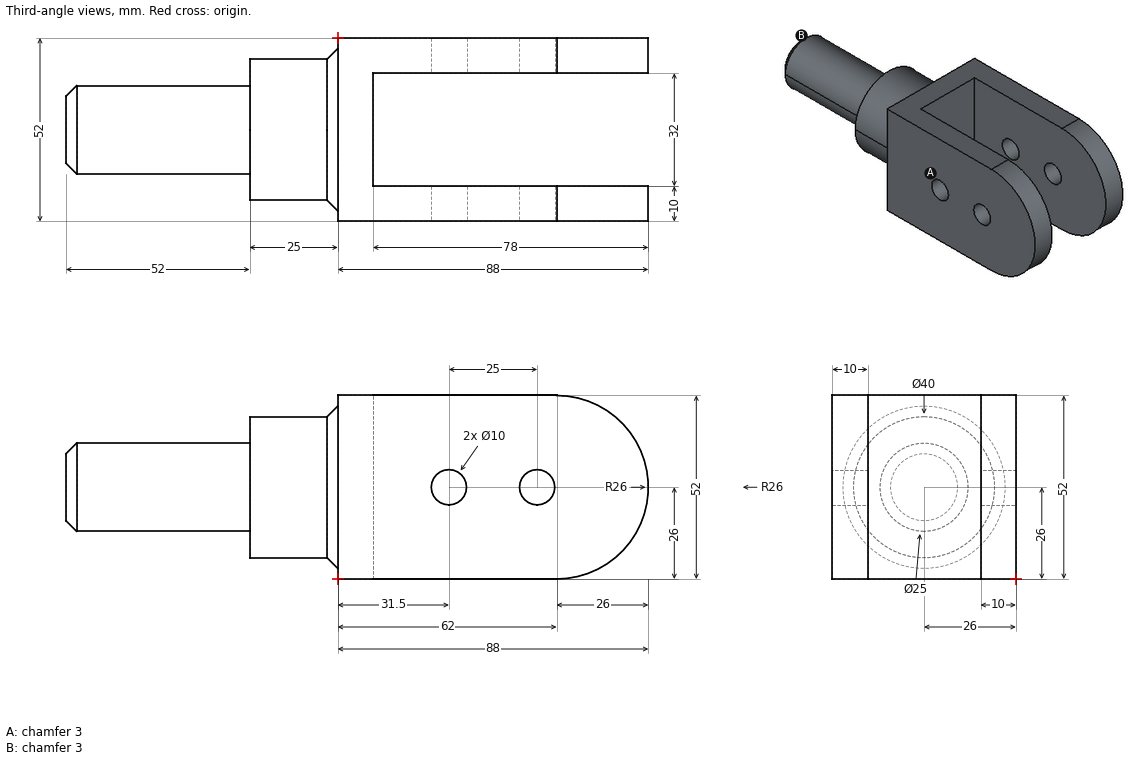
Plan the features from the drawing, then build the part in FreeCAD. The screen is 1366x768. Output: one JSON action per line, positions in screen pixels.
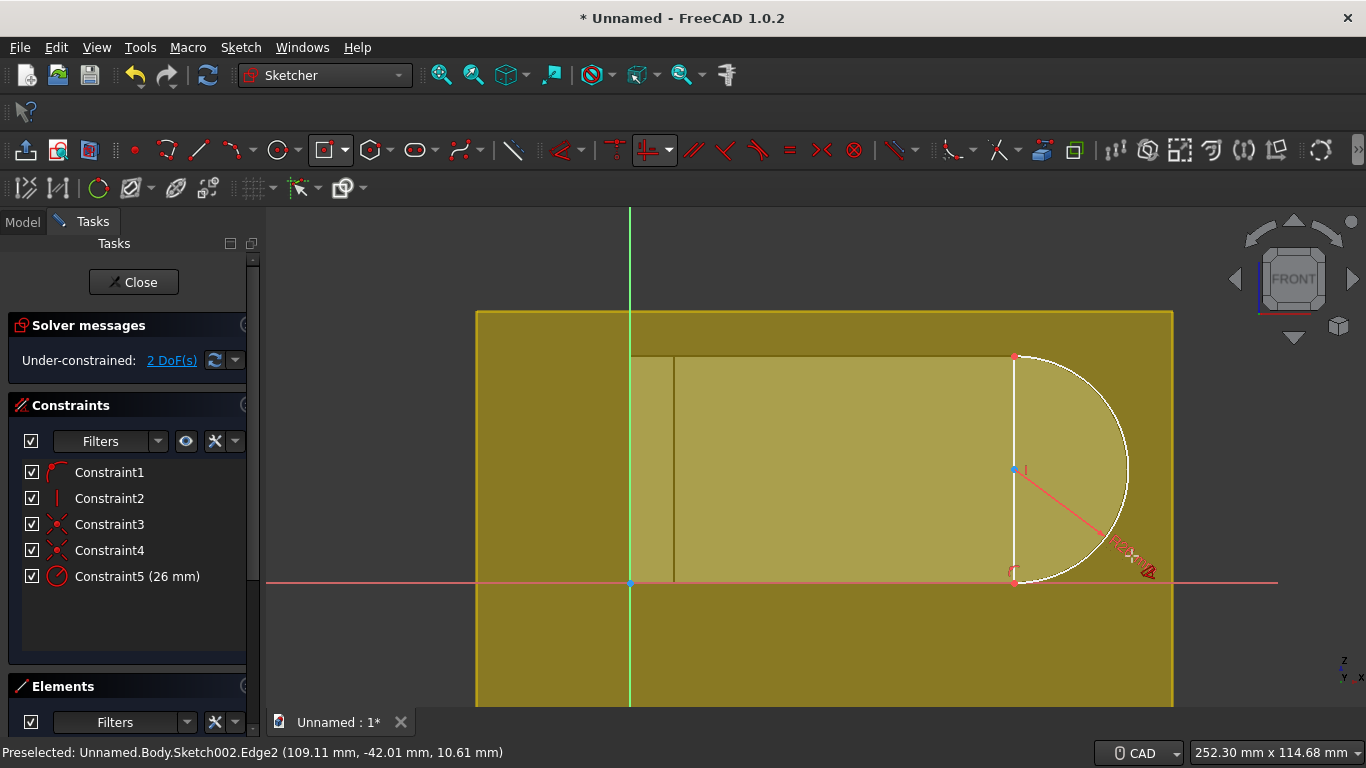
{"action": "left_click", "coordinate": [1014, 356]}
{"action": "left_click", "coordinate": [822, 617]}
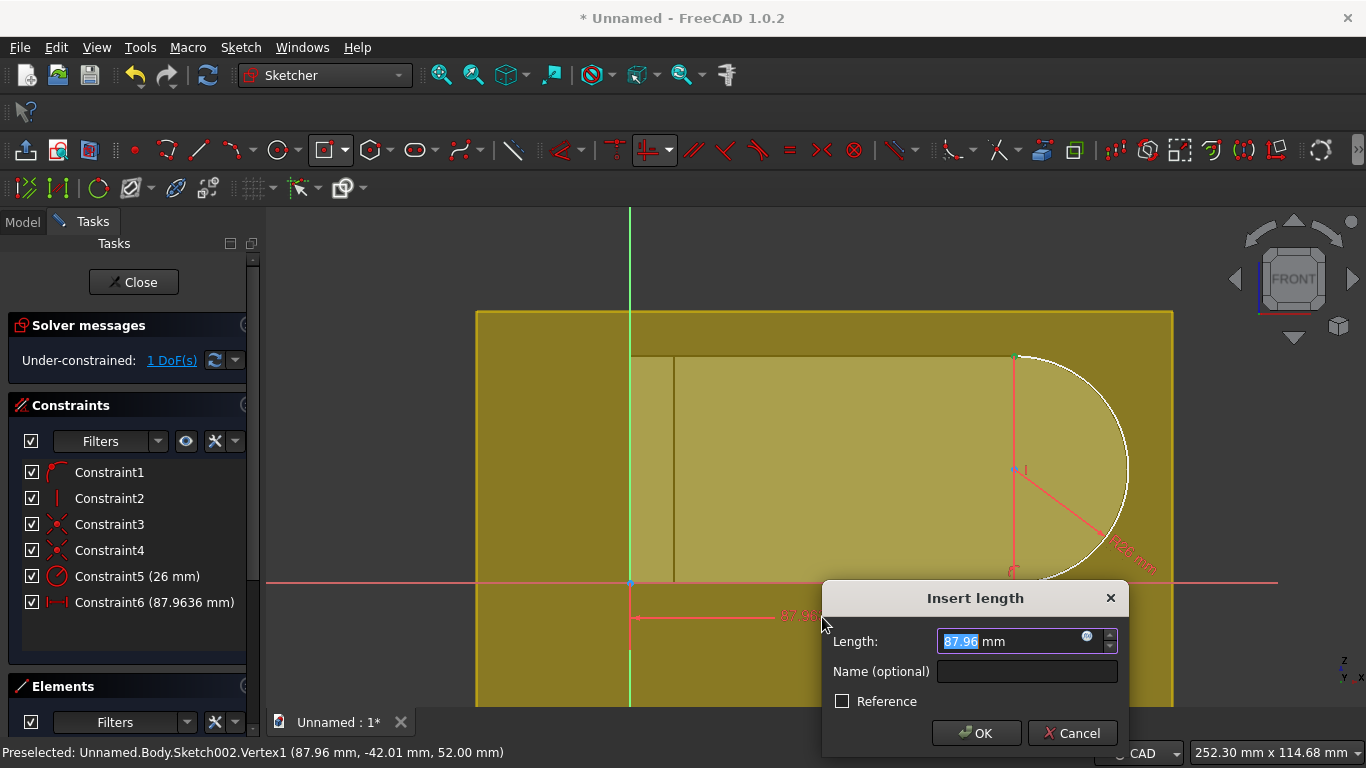
{"action": "type", "text": "88"}
{"action": "key", "text": "Return"}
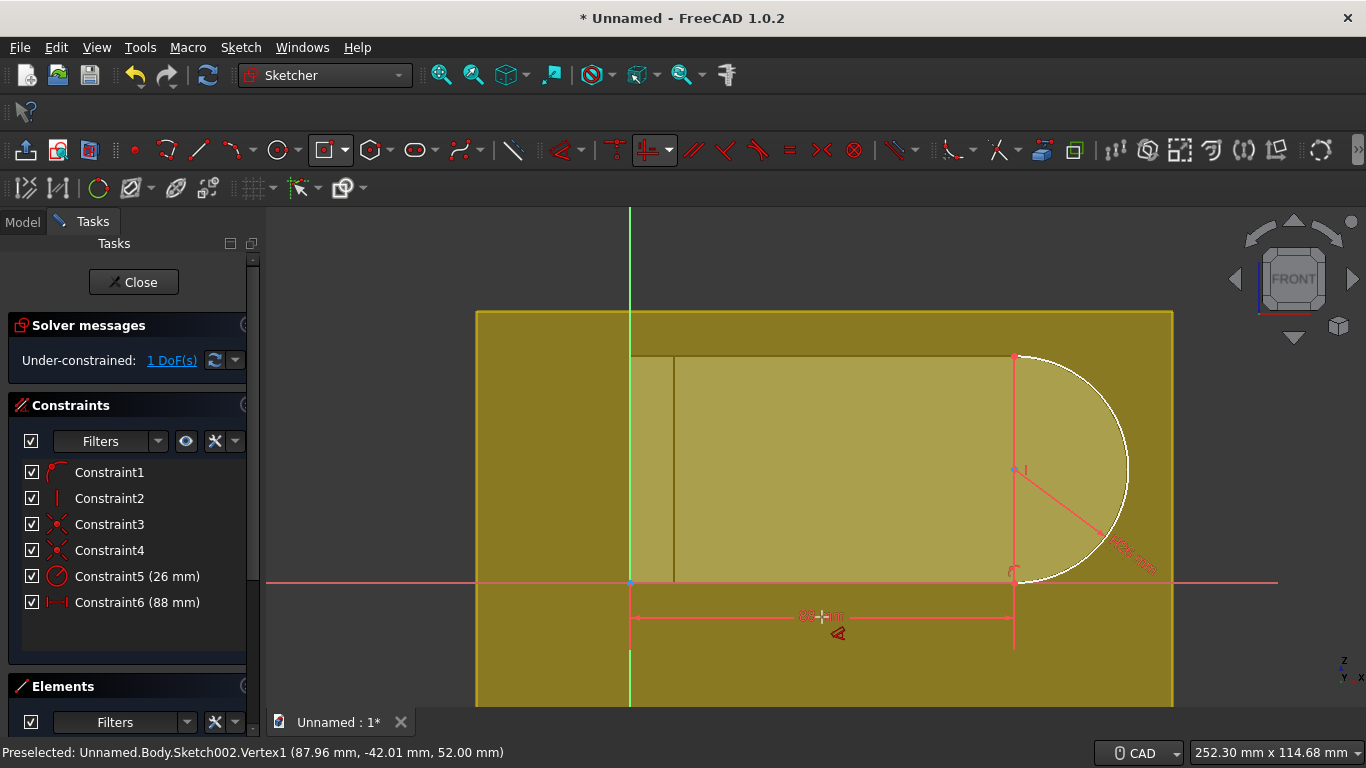
{"action": "left_click", "coordinate": [1015, 470]}
{"action": "left_click", "coordinate": [734, 617]}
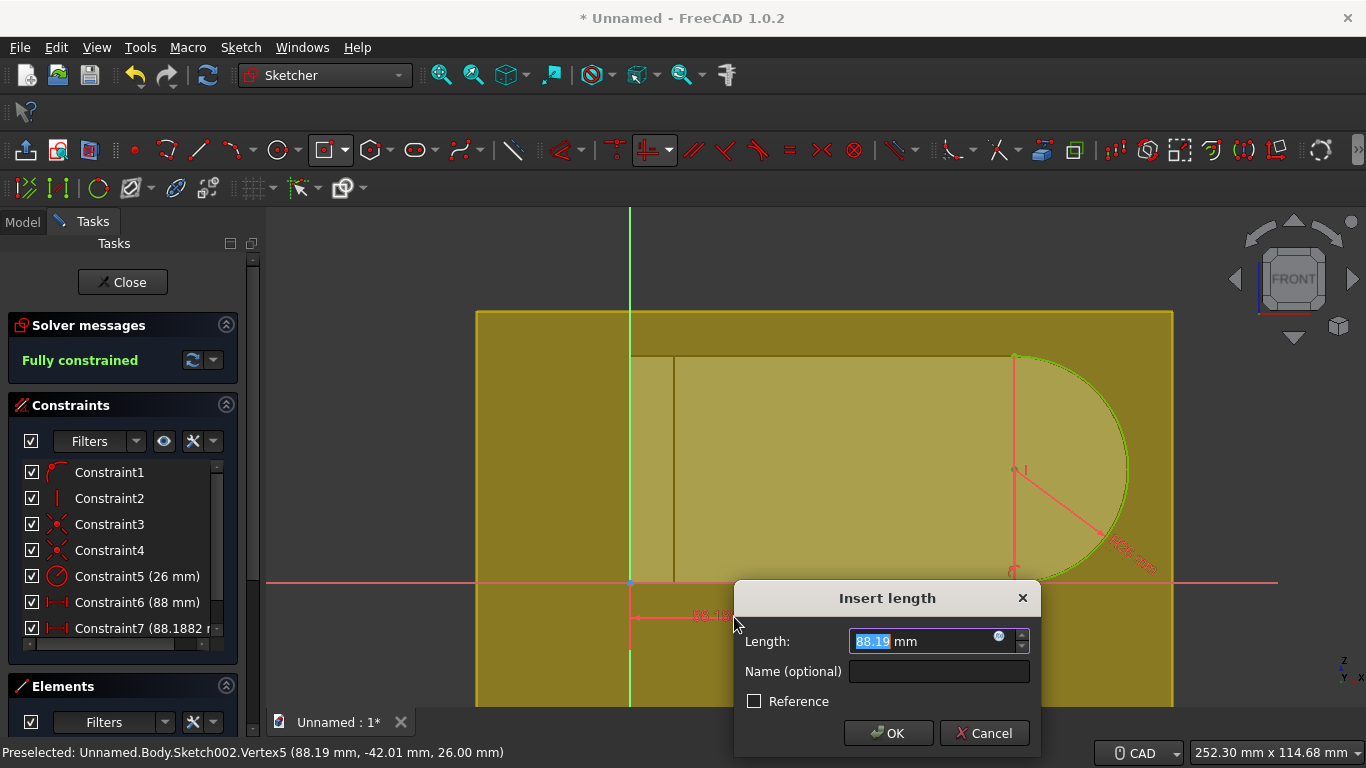
{"action": "type", "text": "88"}
{"action": "key", "text": "Return"}
{"action": "key", "text": "Escape"}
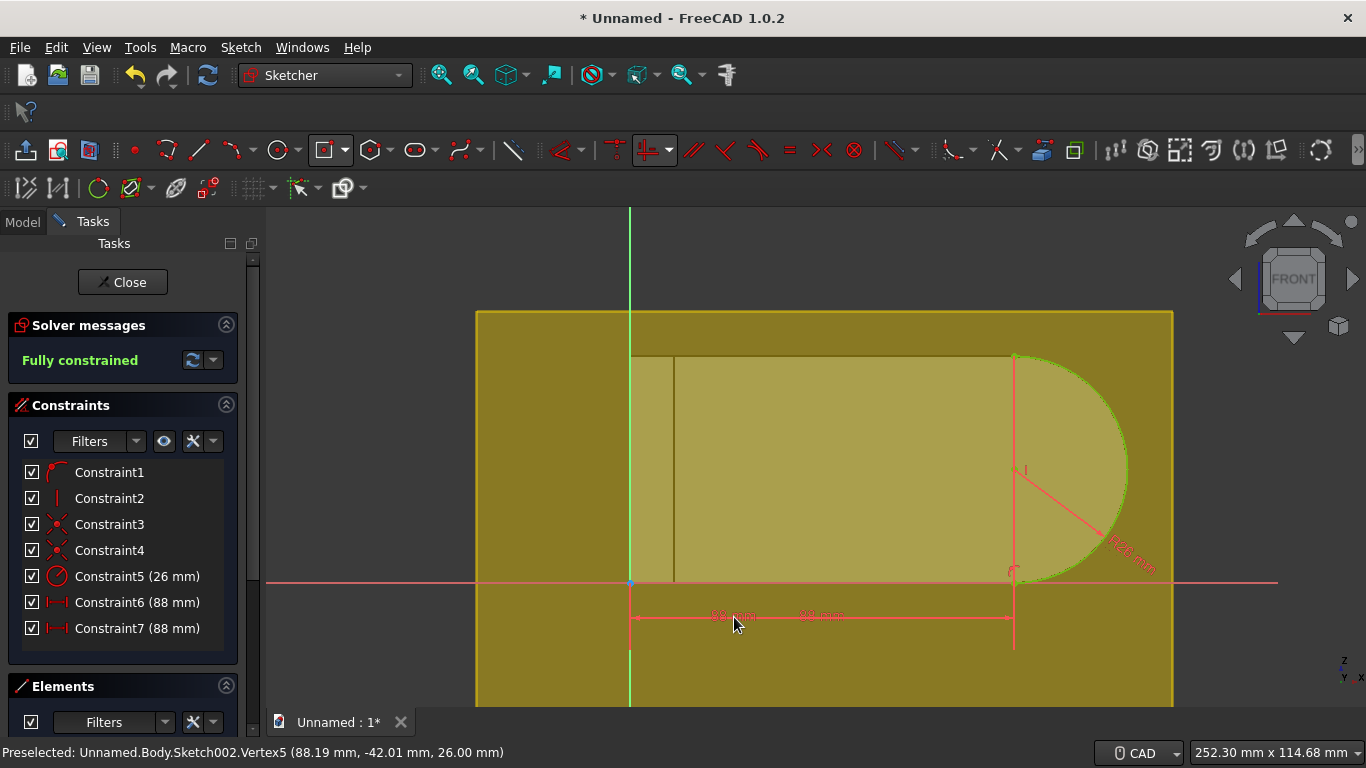
{"action": "left_click", "coordinate": [123, 282]}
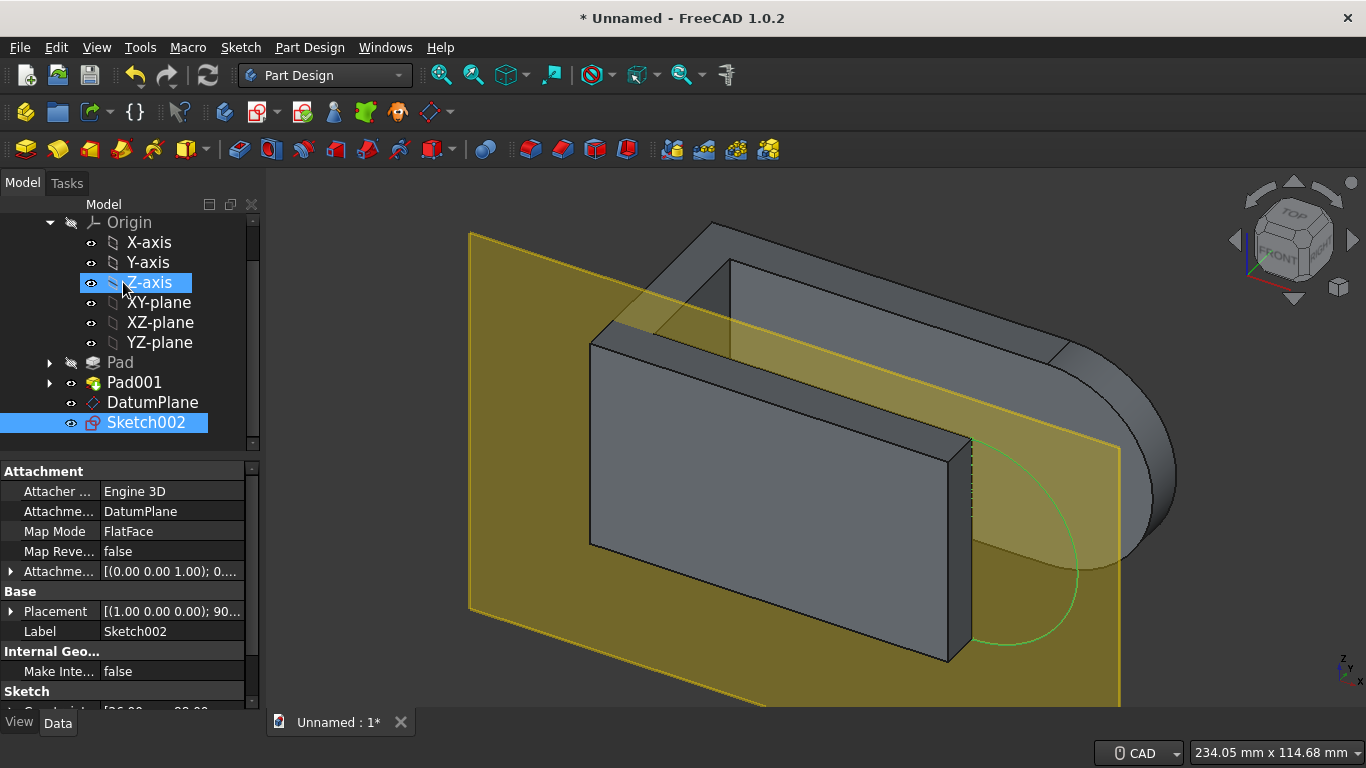
{"action": "left_click", "coordinate": [26, 150]}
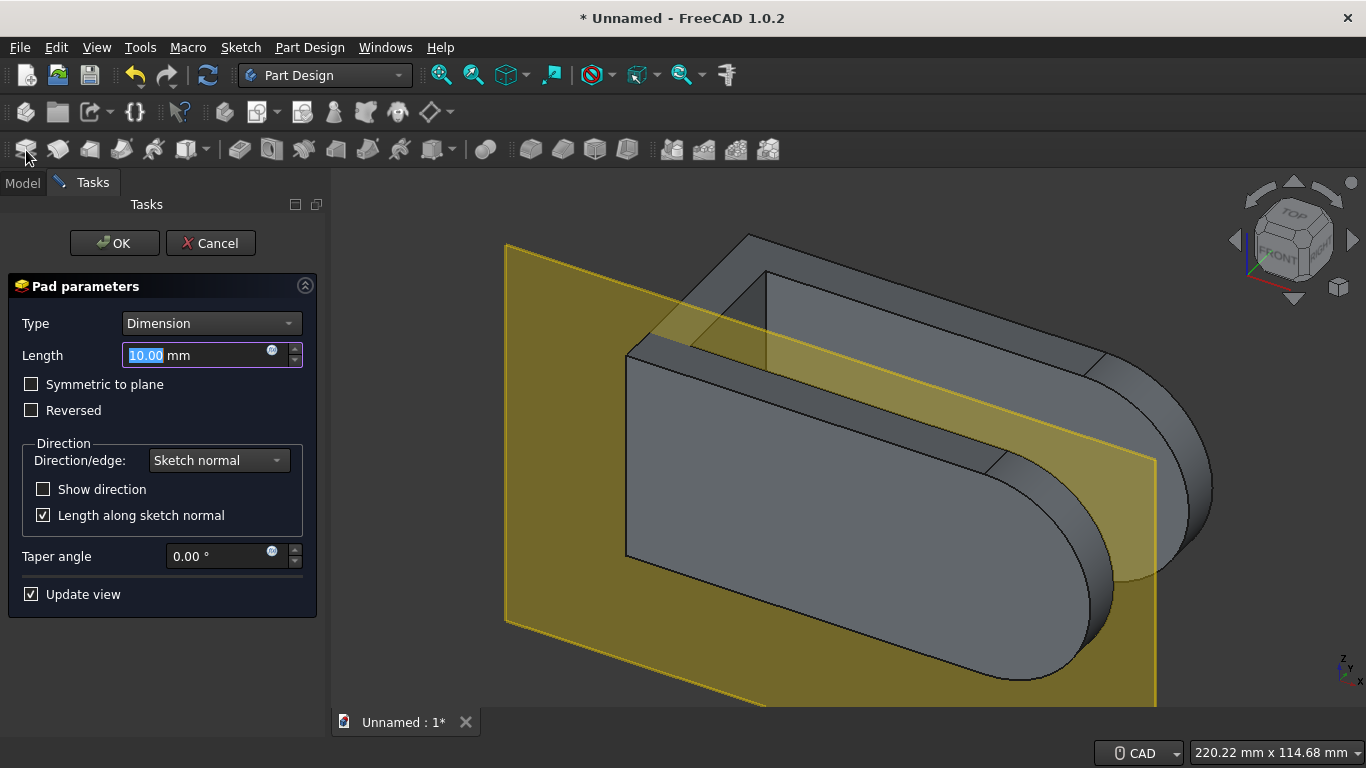
{"action": "type", "text": "10"}
{"action": "key", "text": "Tab"}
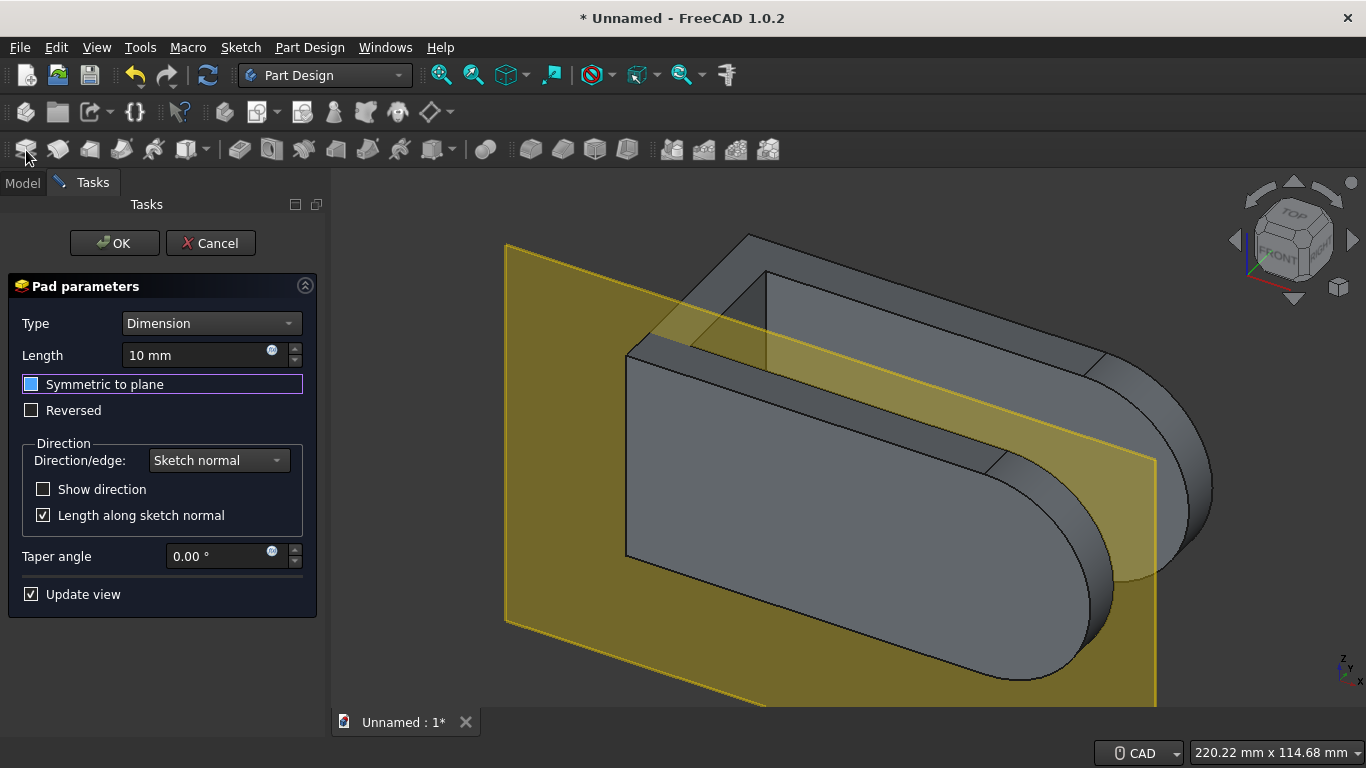
{"action": "left_click", "coordinate": [115, 243]}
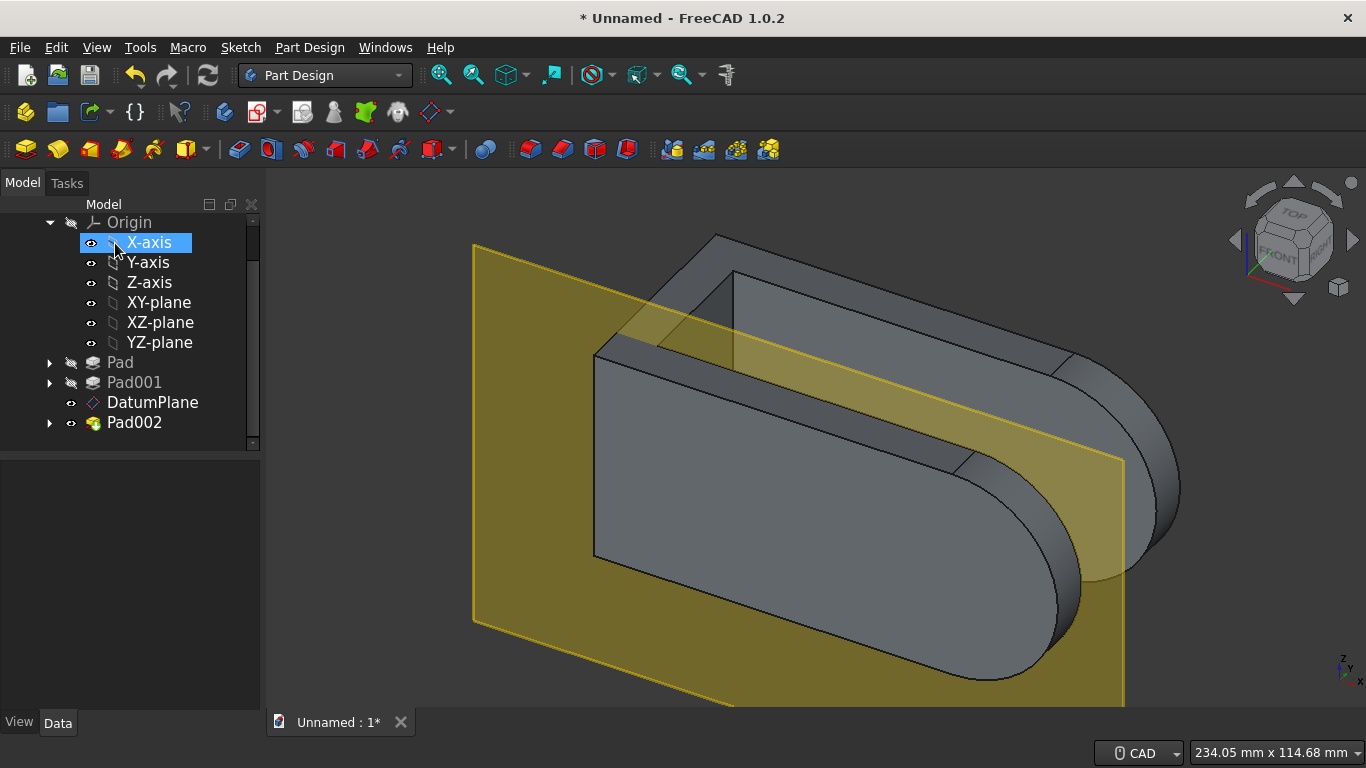
{"action": "left_click", "coordinate": [116, 403]}
{"action": "key", "text": "space"}